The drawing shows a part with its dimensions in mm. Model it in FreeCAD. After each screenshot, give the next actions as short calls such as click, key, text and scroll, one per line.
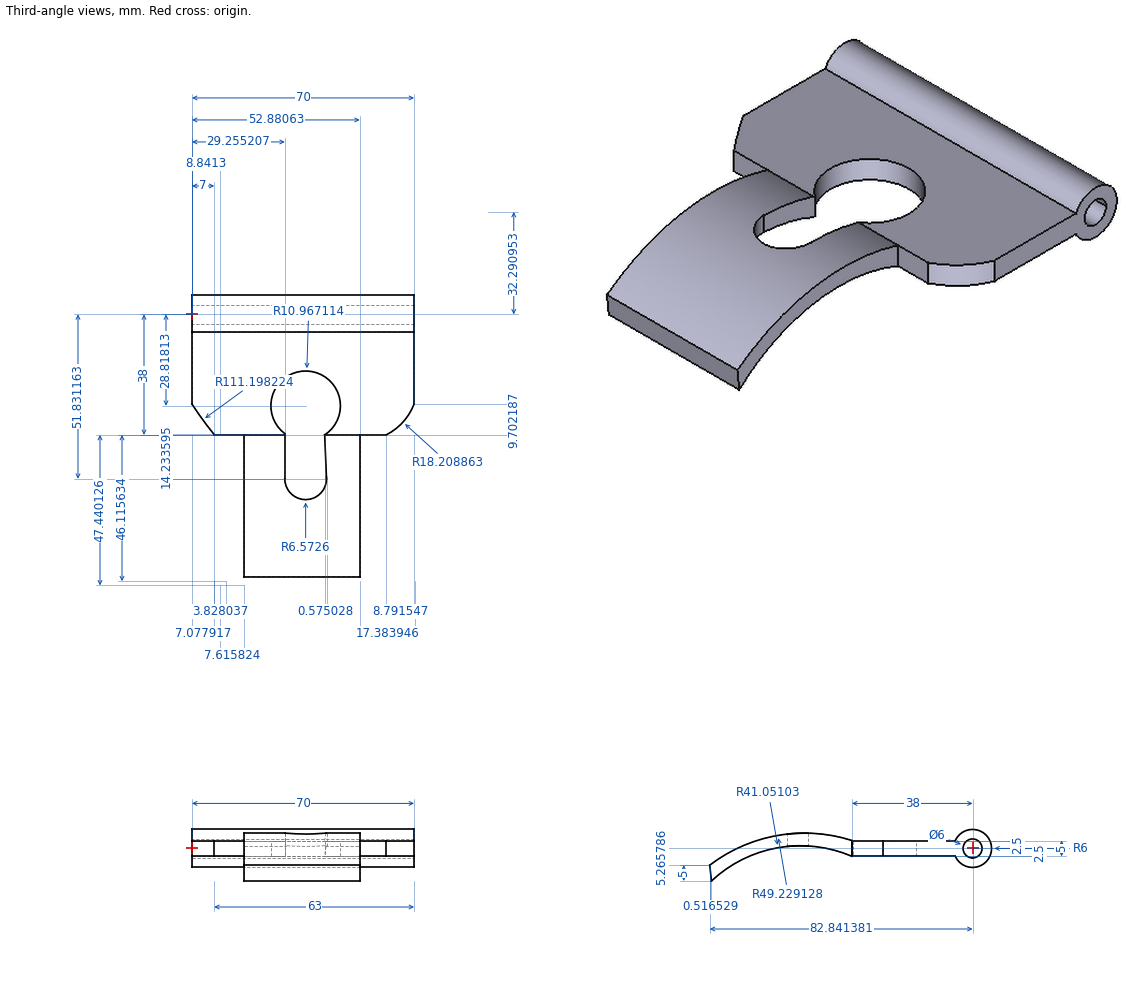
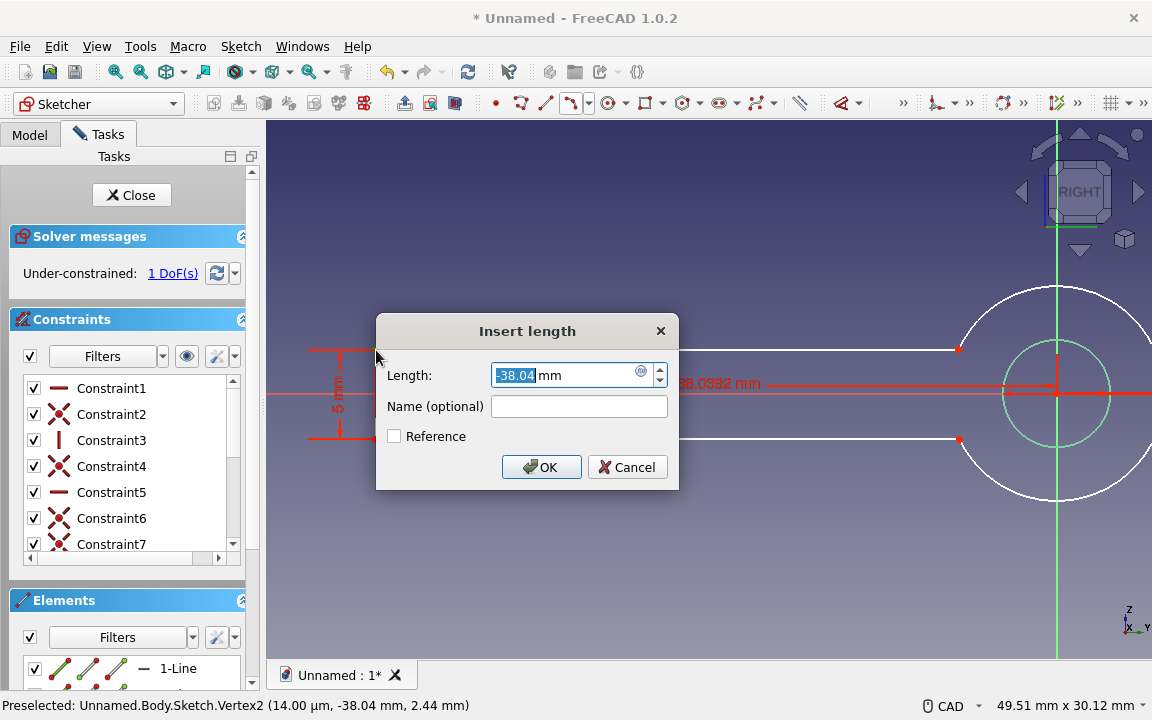
text(-38)
key(Return)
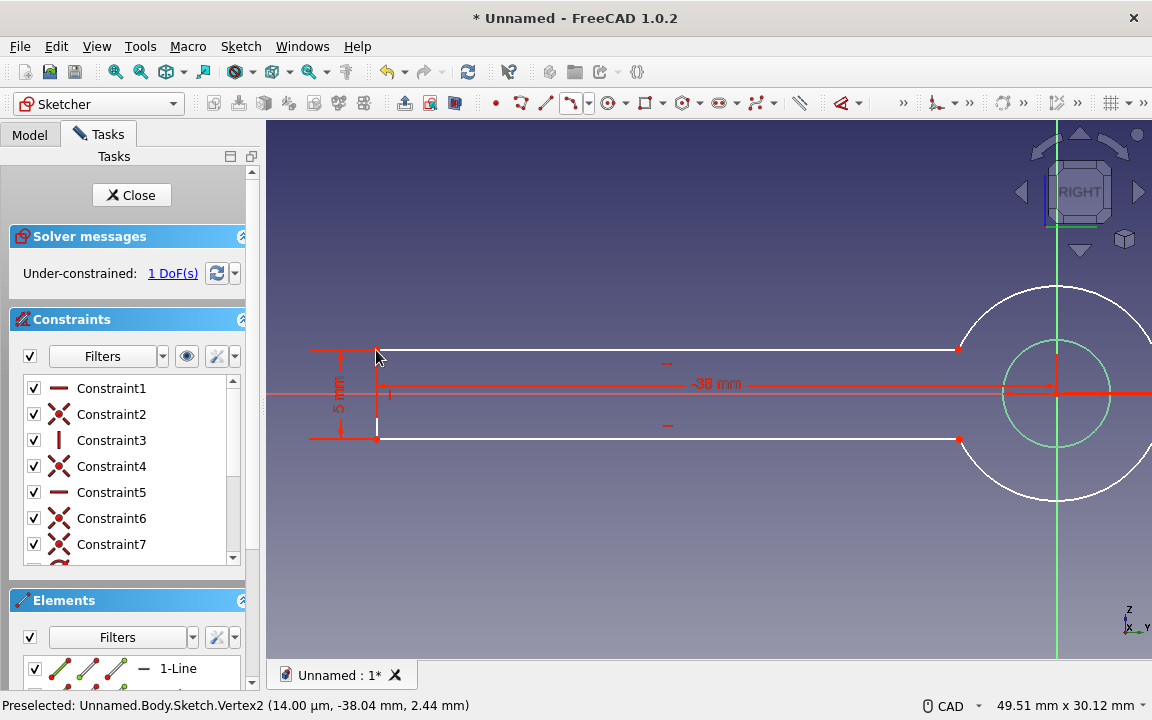
click(959, 350)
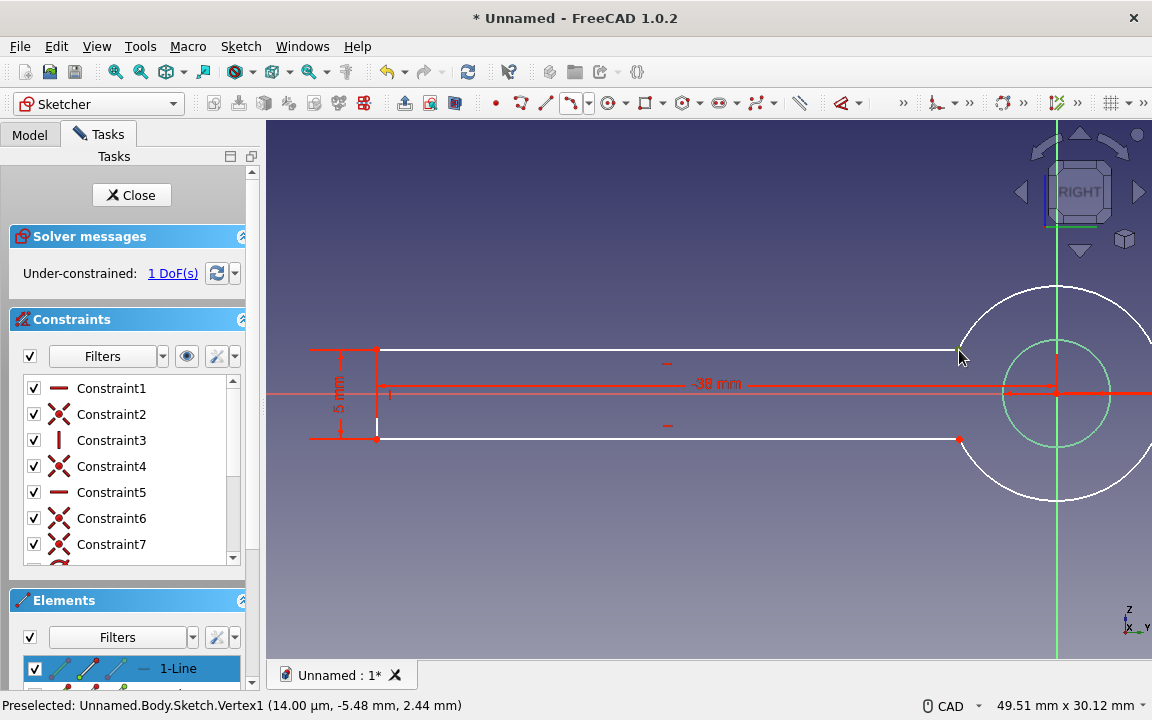
click(858, 104)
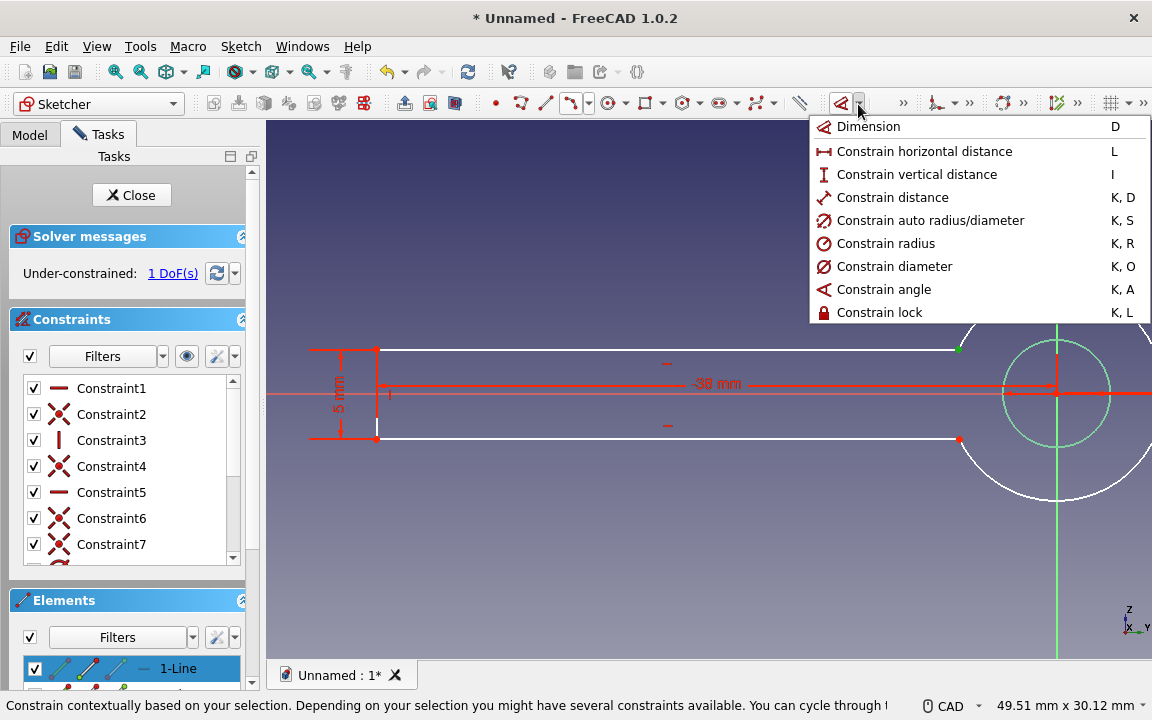
click(980, 174)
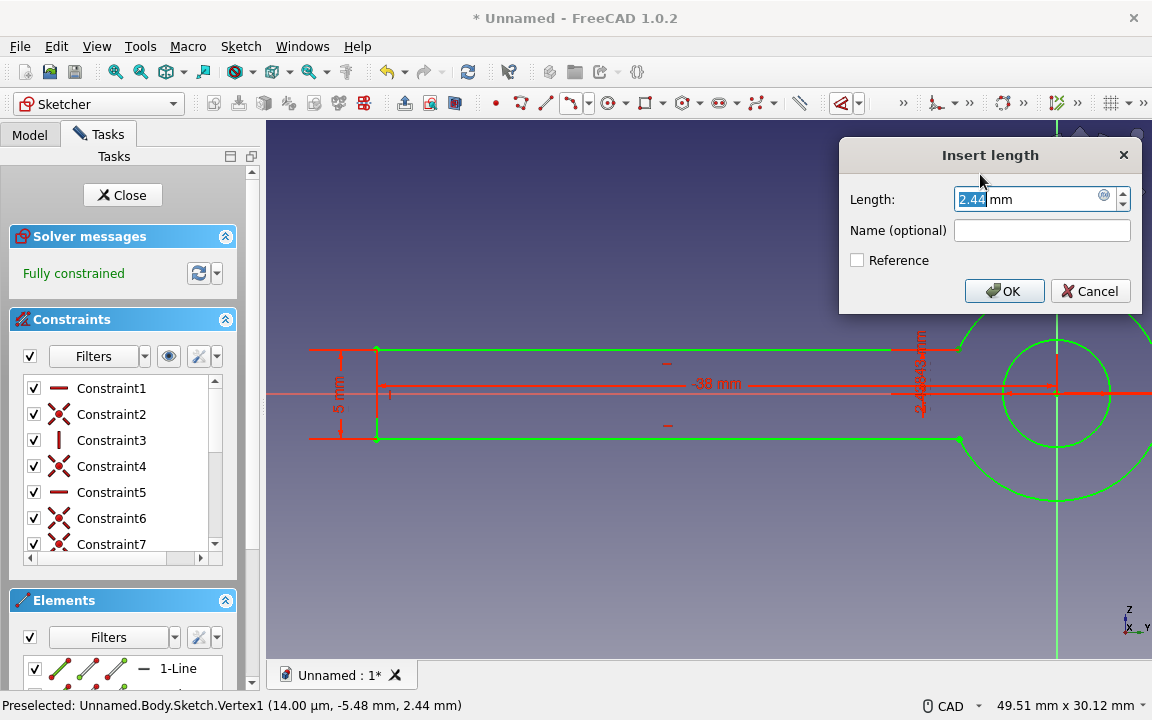
text(2.5)
key(Return)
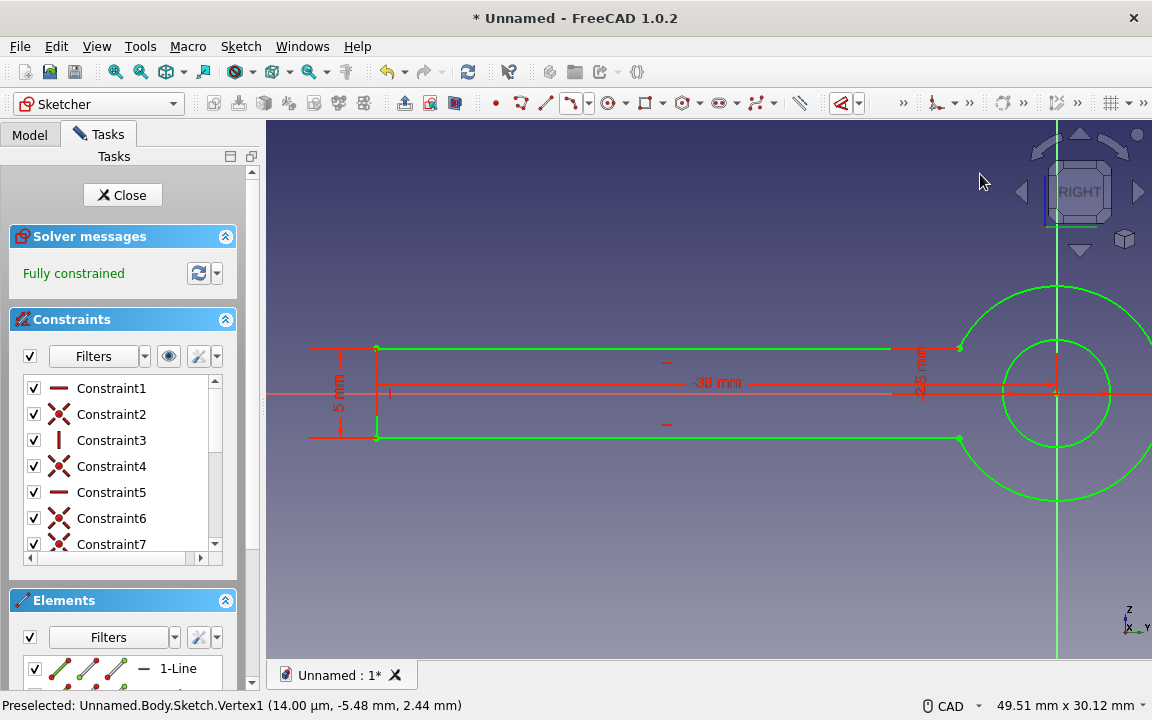
click(123, 195)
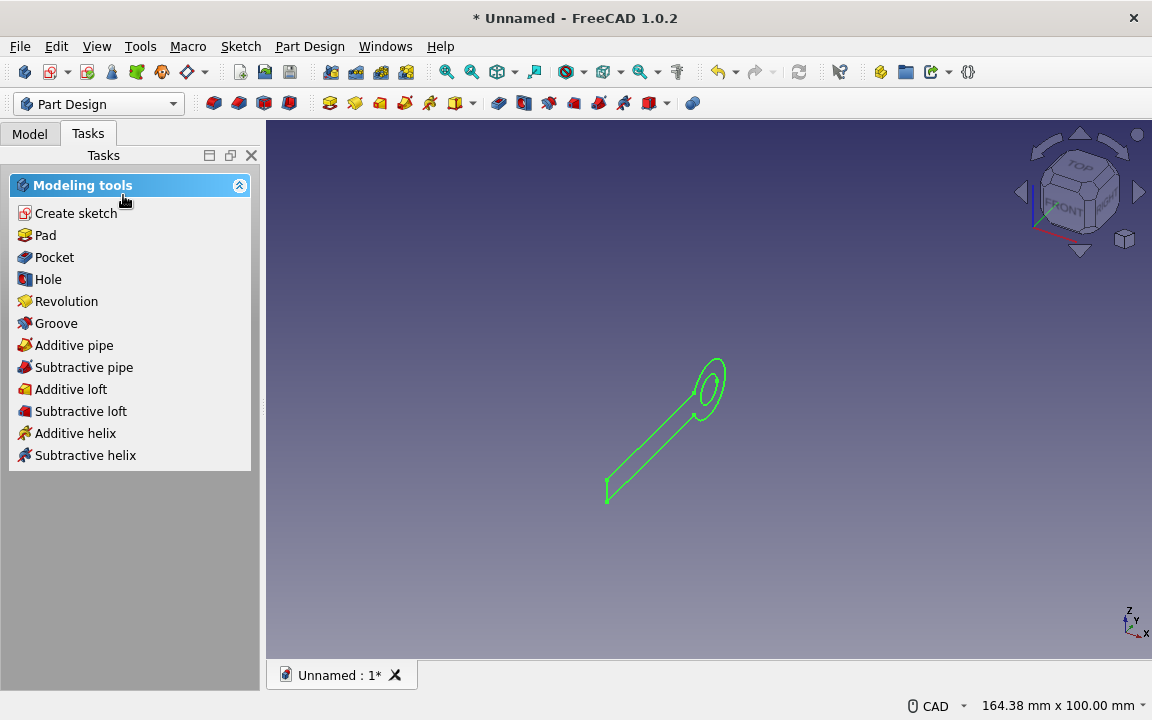
click(330, 104)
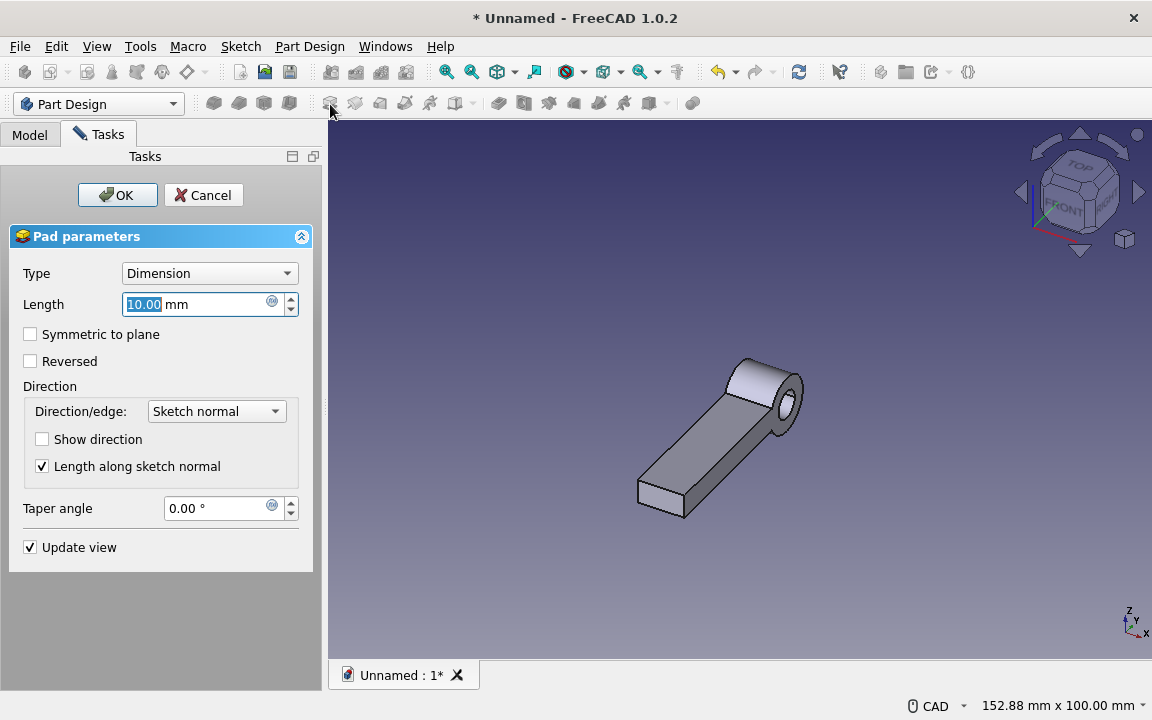
text(70)
key(Tab)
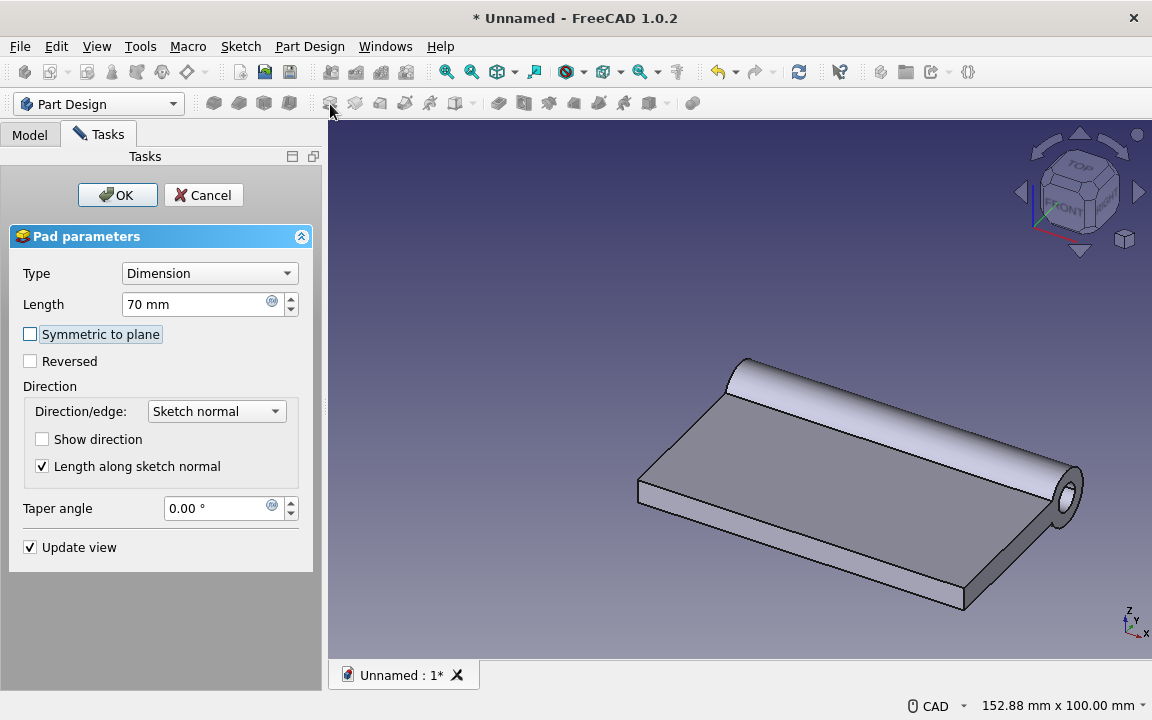
click(118, 195)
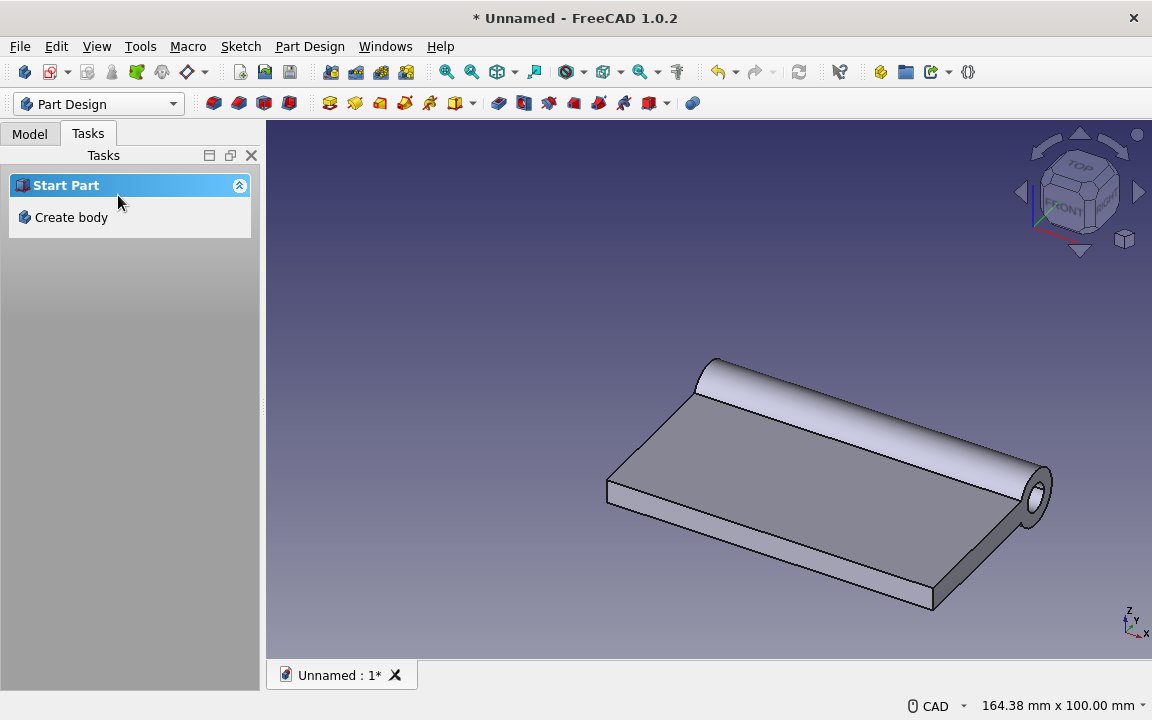
key(5)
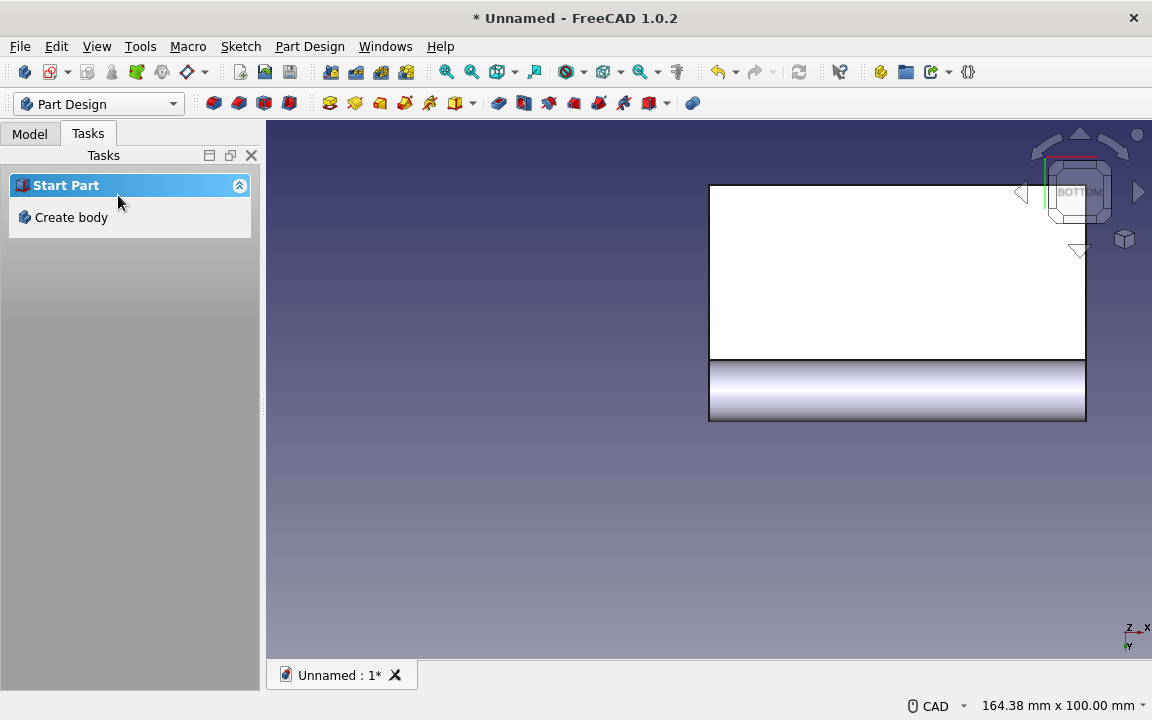
click(447, 72)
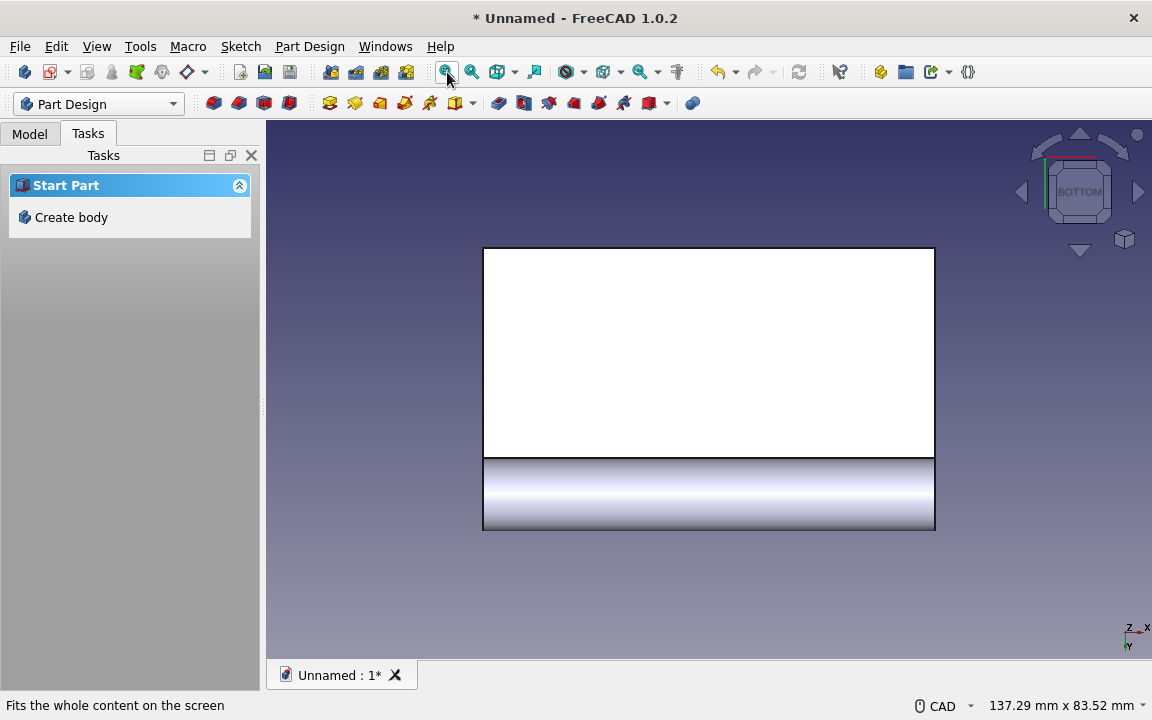
click(774, 352)